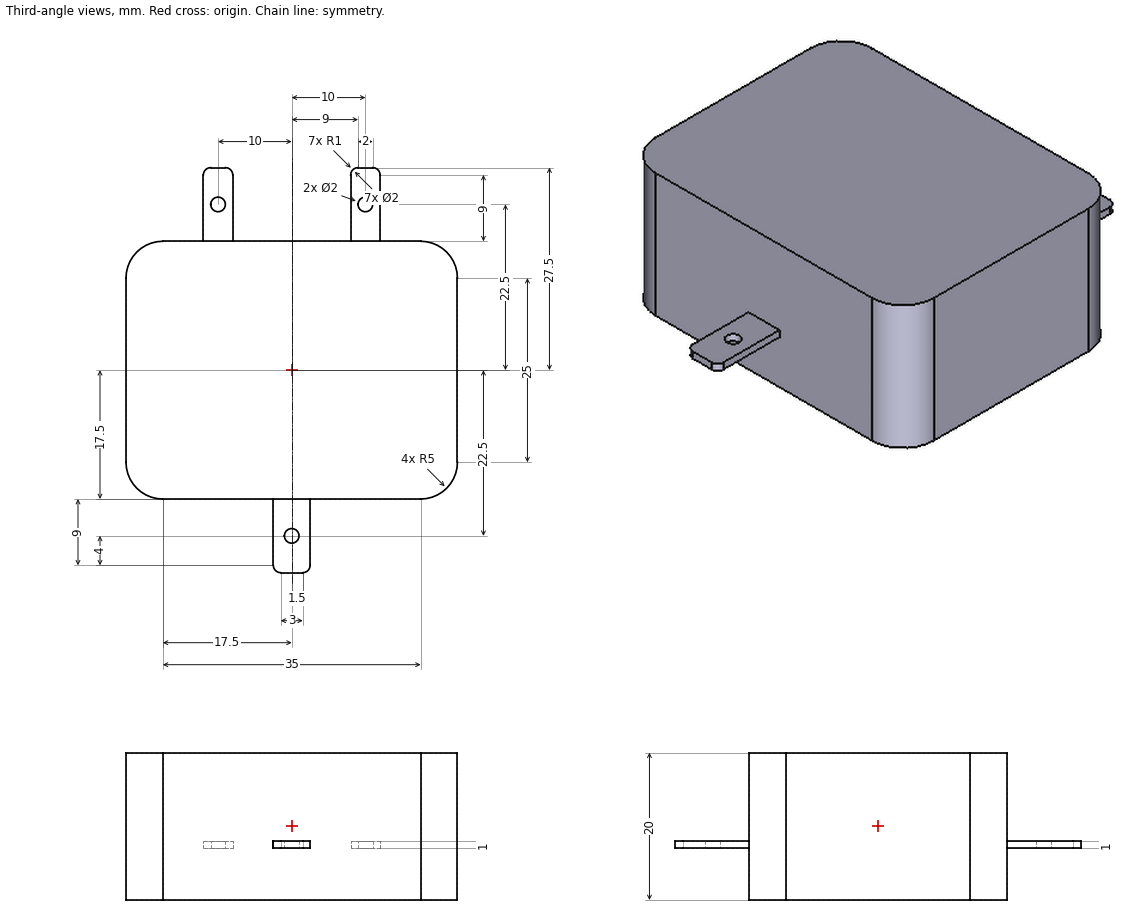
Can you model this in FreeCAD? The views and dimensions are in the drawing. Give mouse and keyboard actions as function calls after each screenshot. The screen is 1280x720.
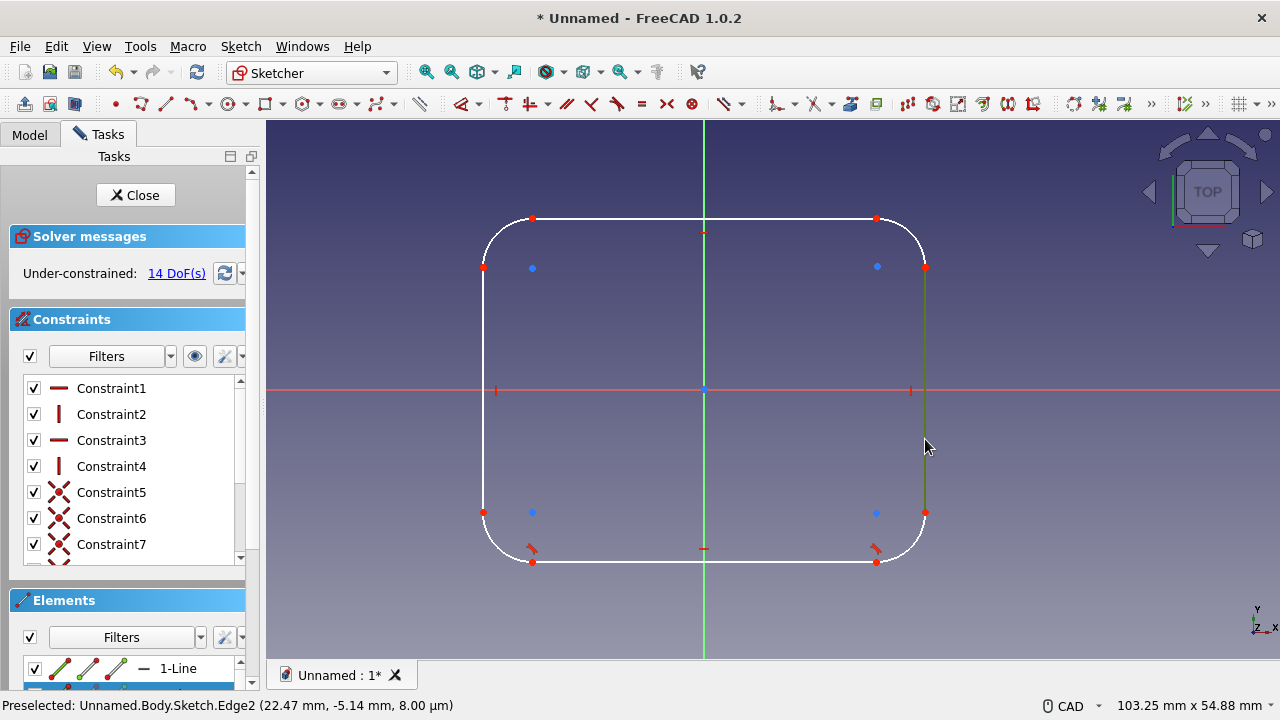
click(898, 557)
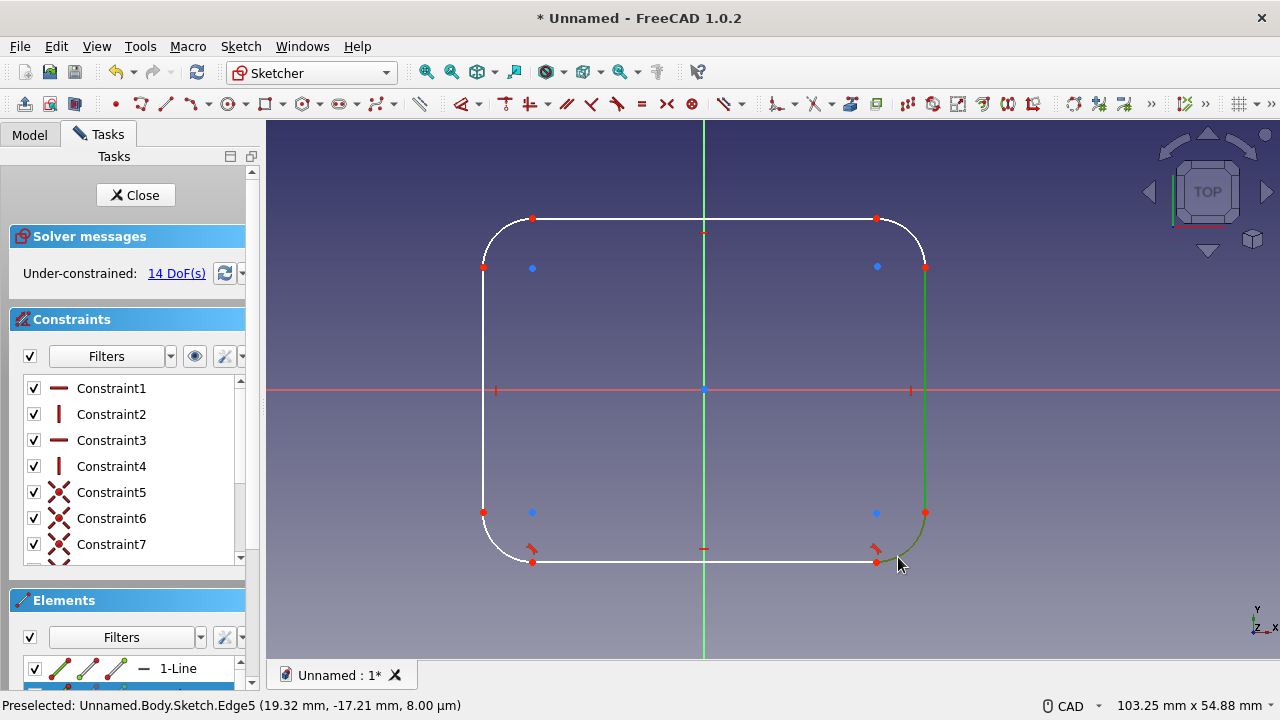
click(617, 104)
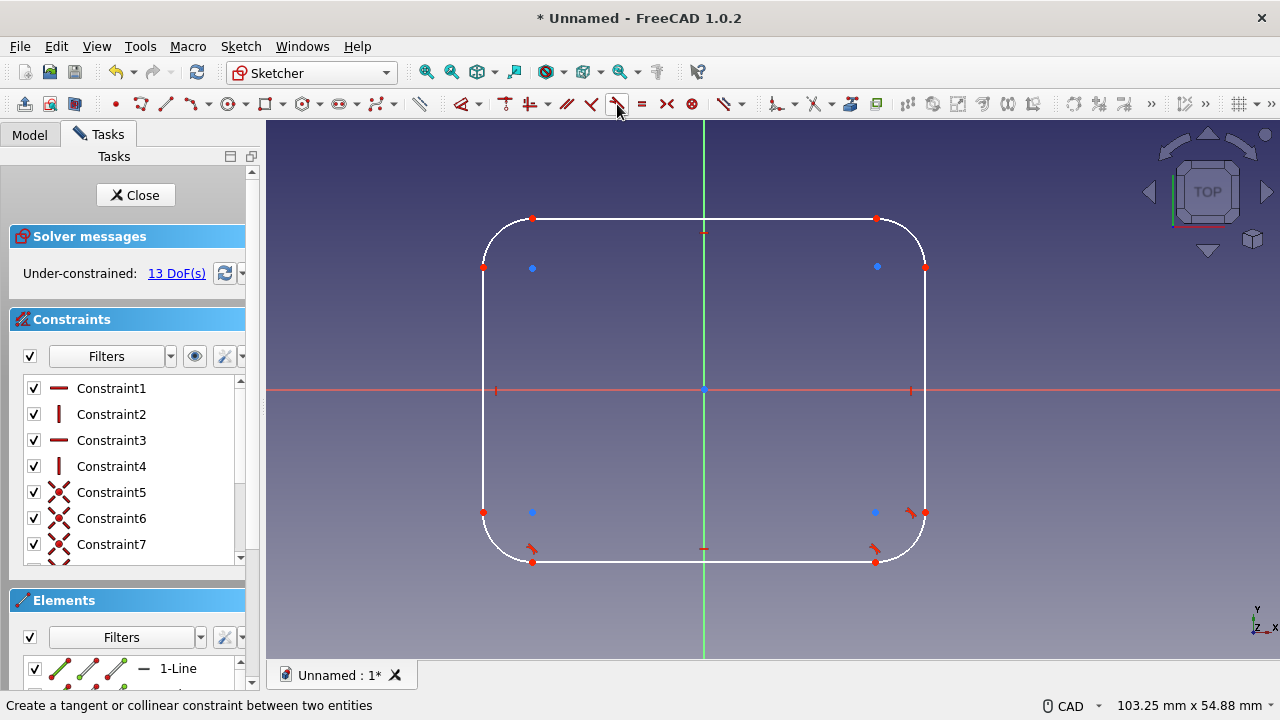
click(925, 439)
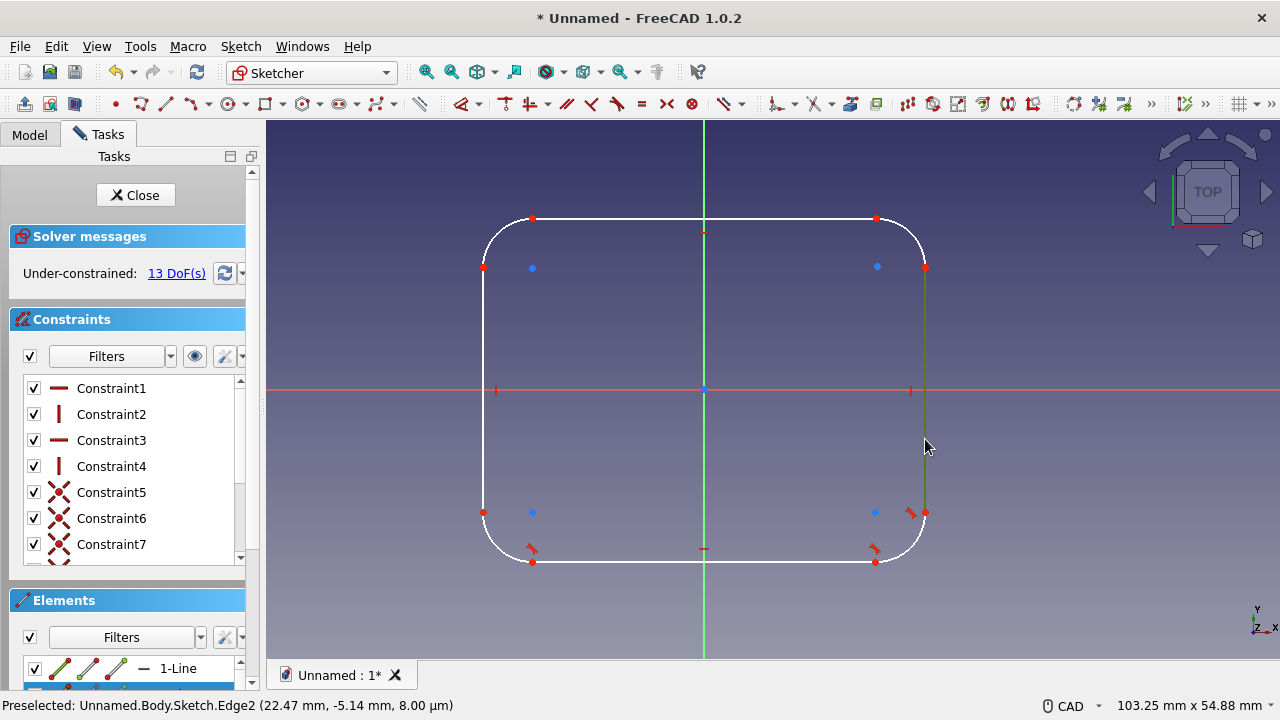
click(920, 246)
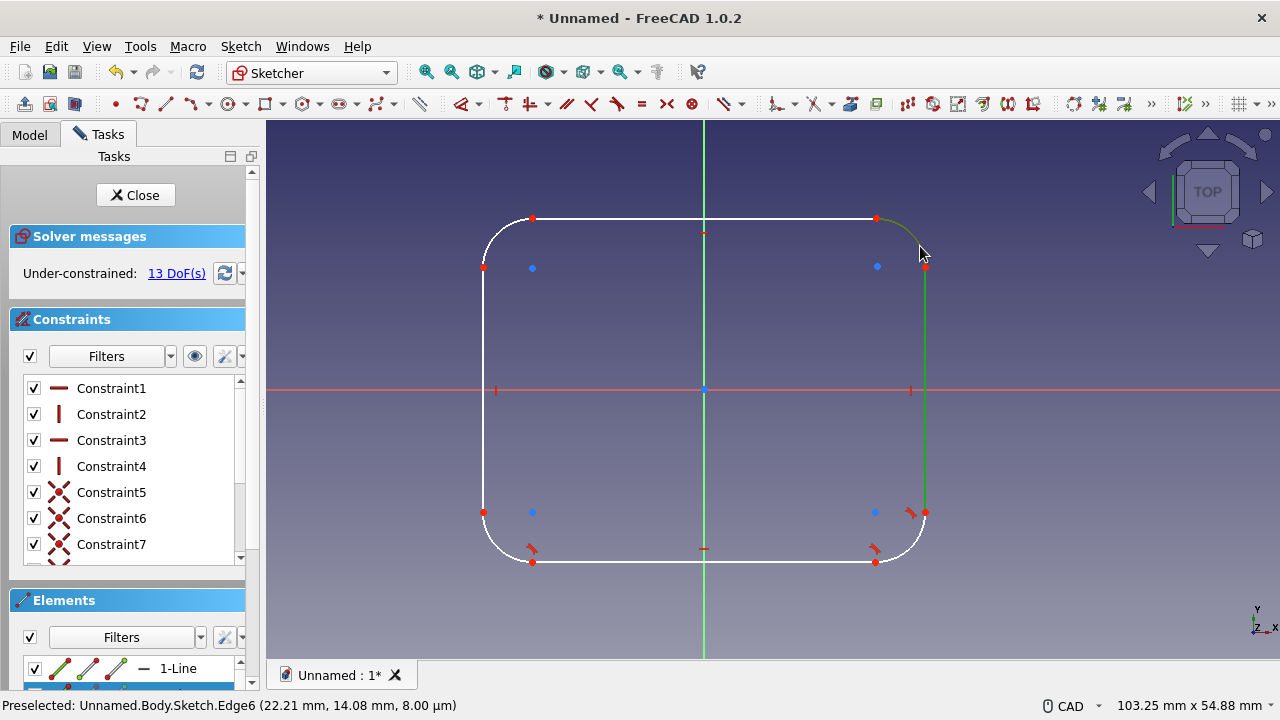
click(617, 104)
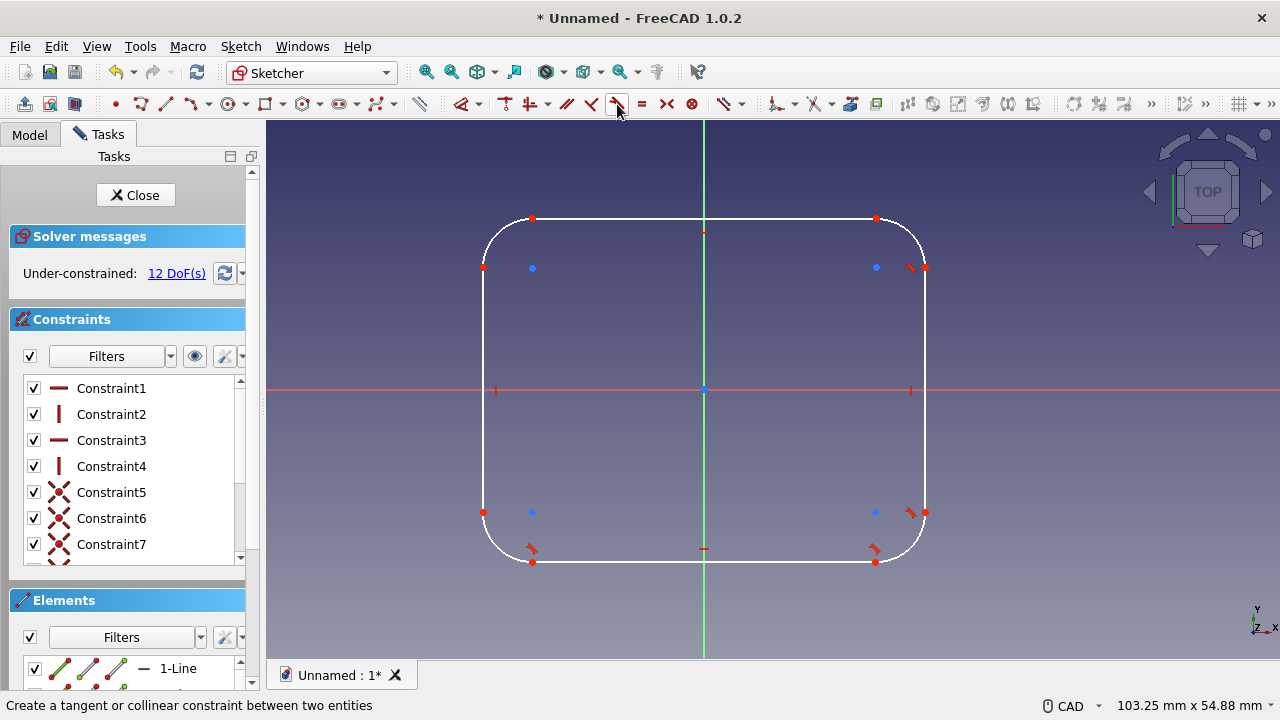
click(773, 219)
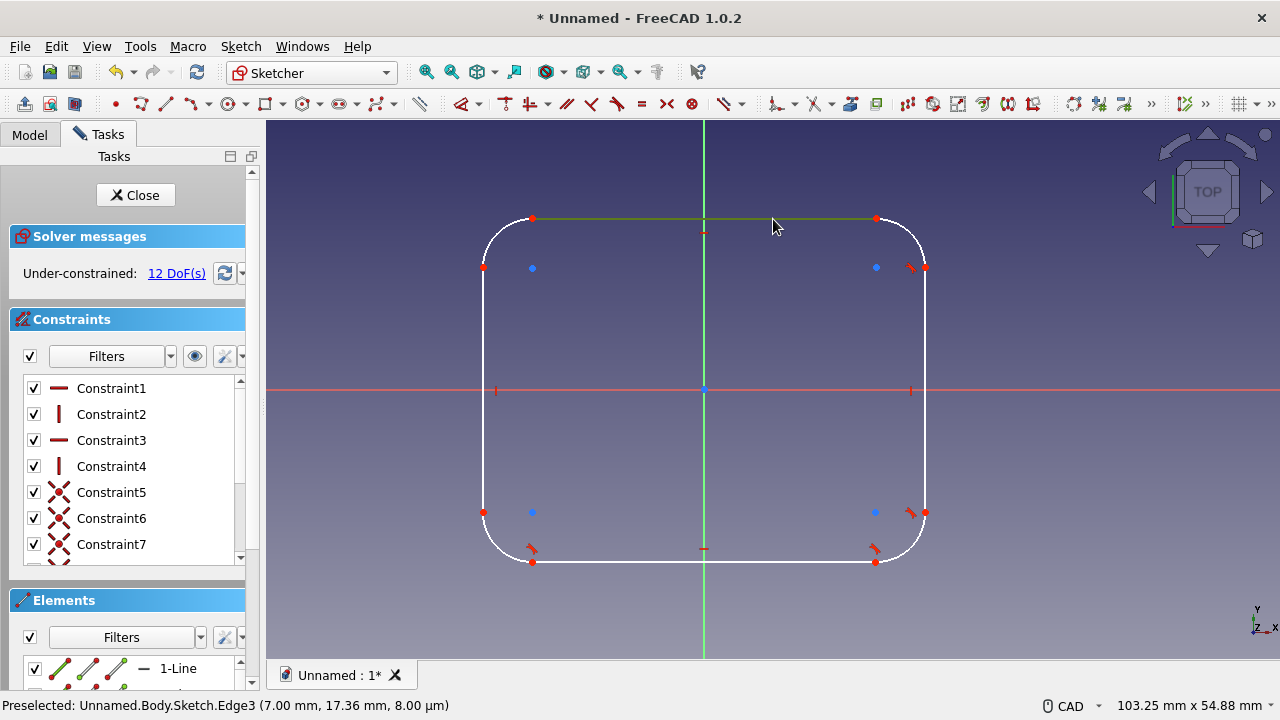
click(920, 246)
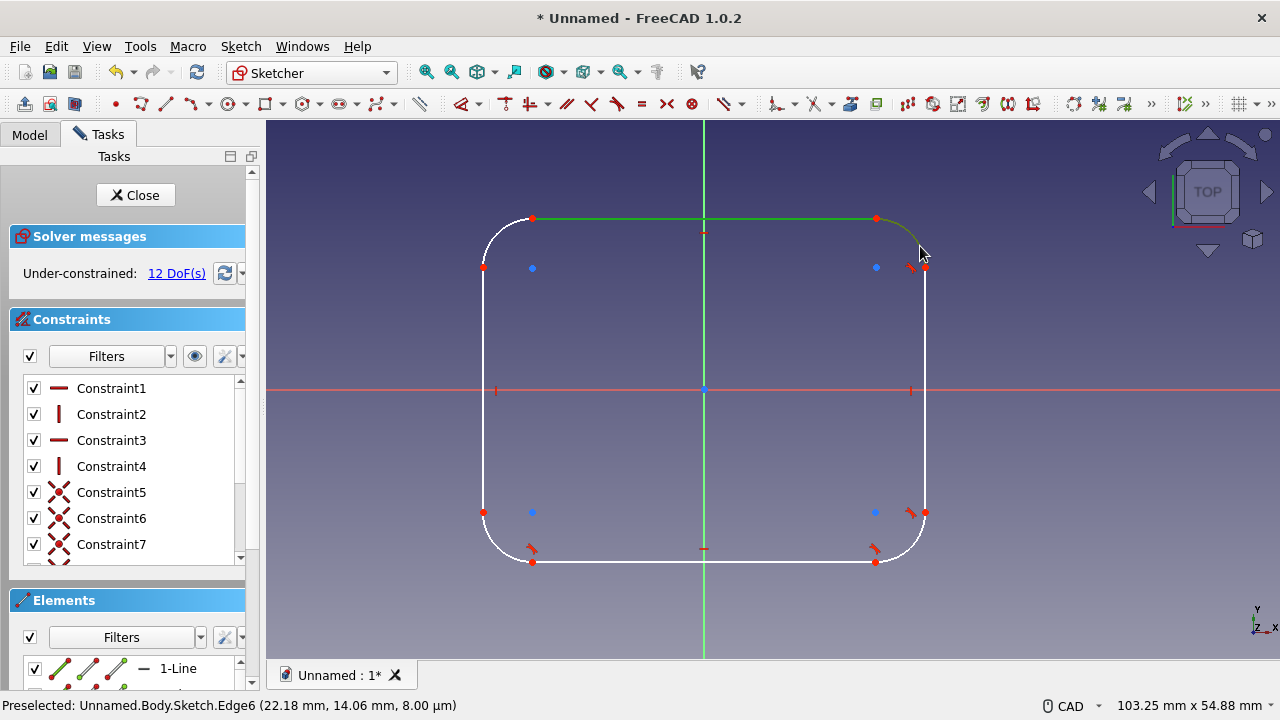
click(617, 104)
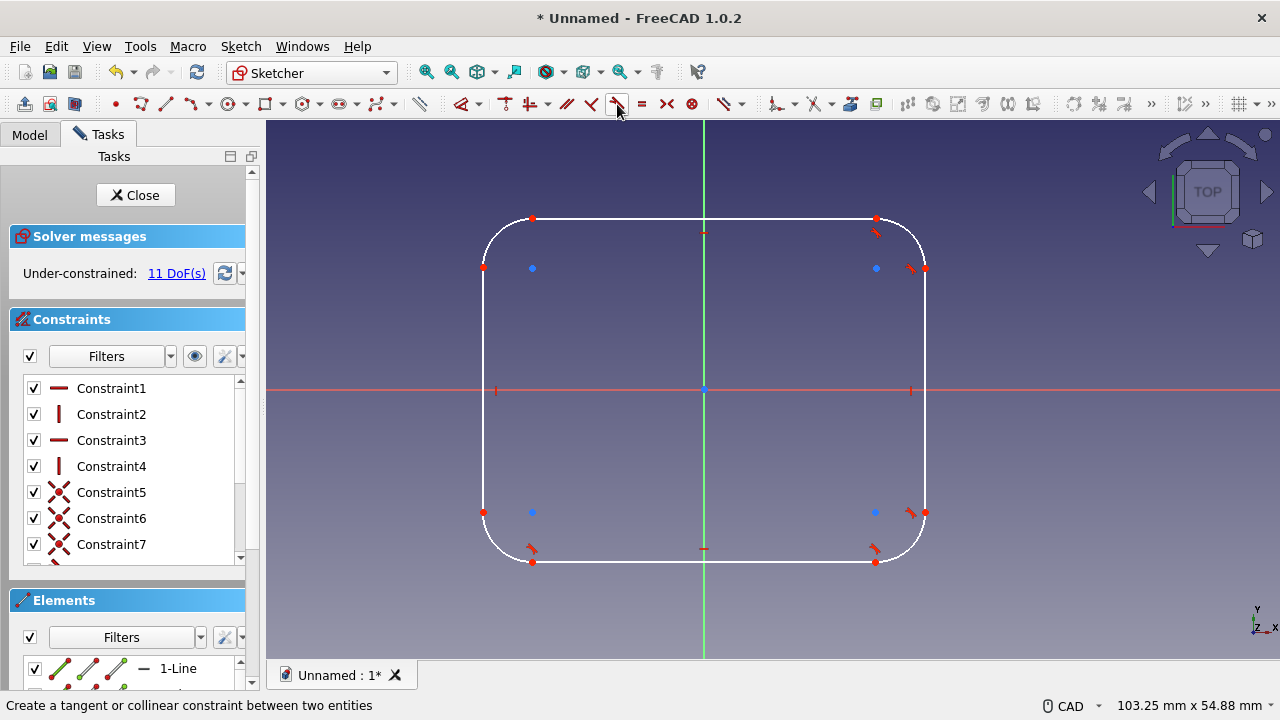
click(773, 219)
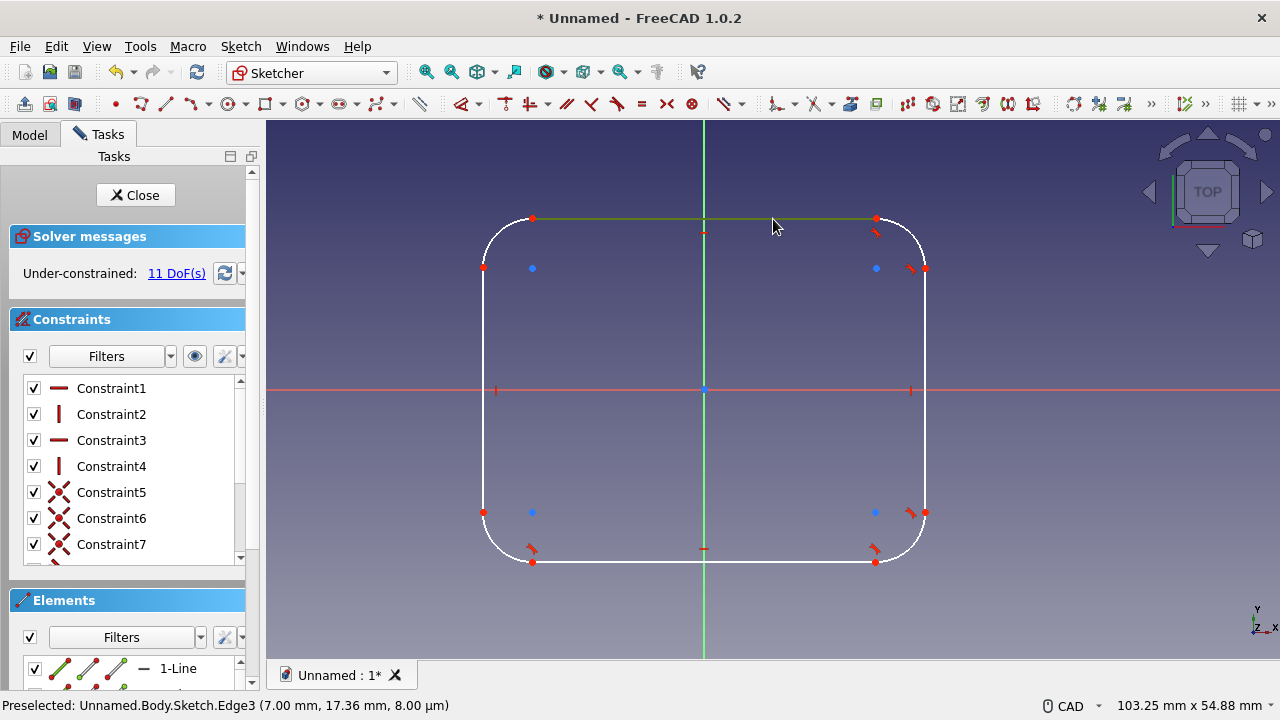
click(510, 224)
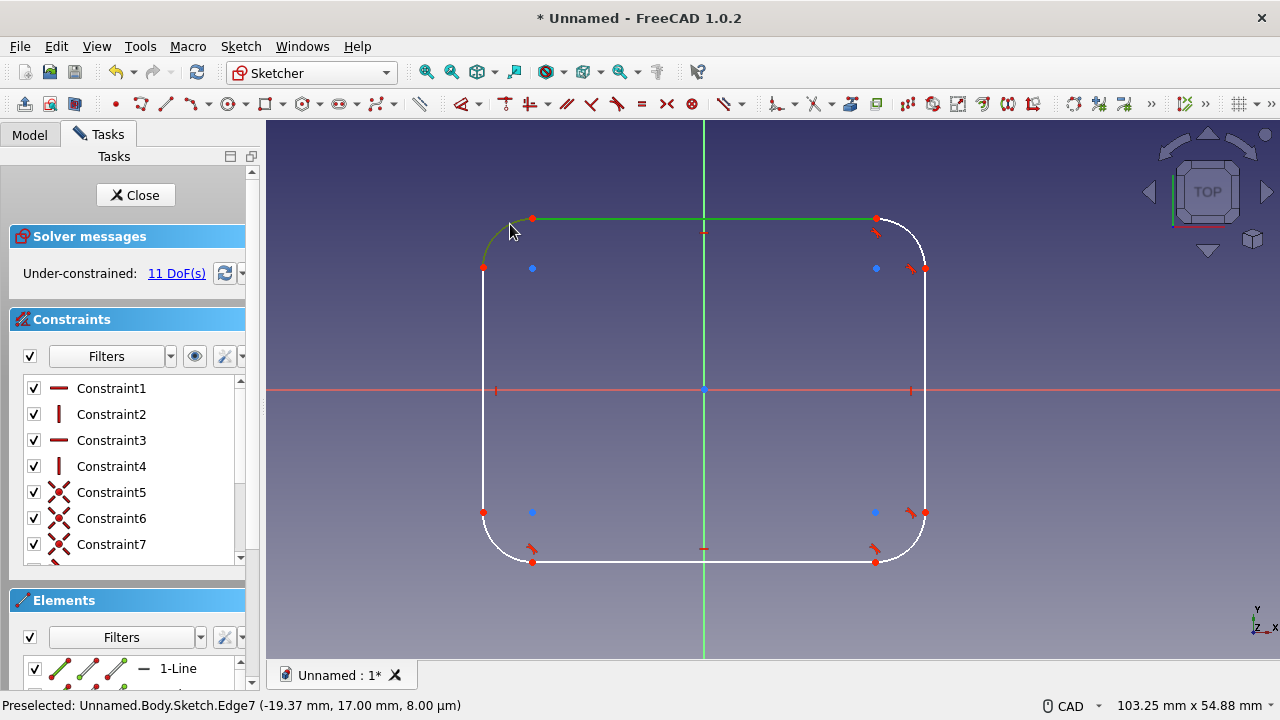
click(617, 104)